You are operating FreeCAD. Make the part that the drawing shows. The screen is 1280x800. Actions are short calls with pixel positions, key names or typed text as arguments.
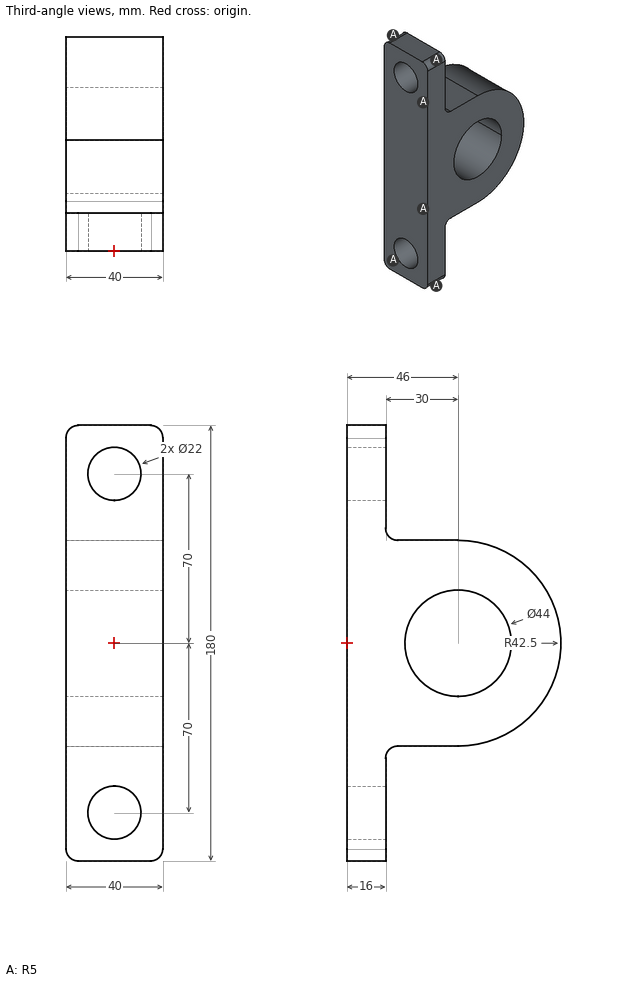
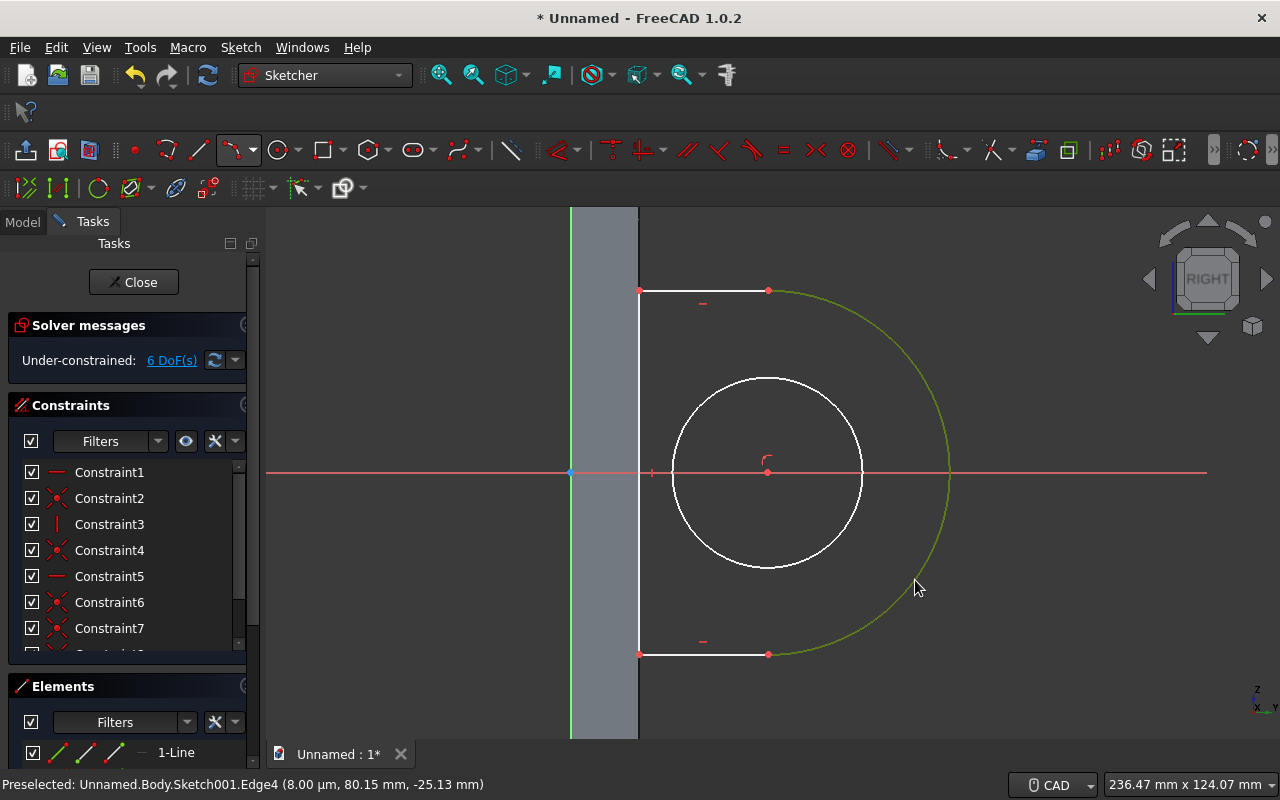
key(k)
key(r)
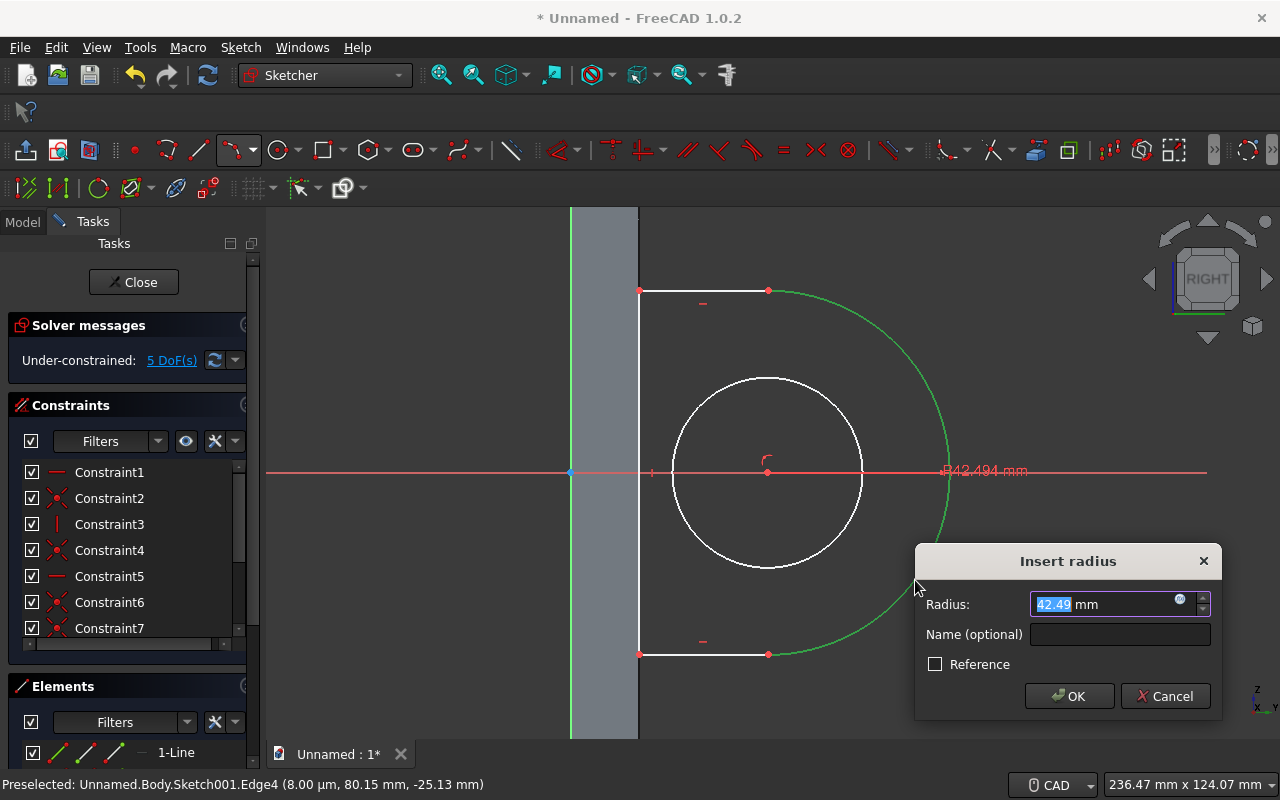
text(42.5)
key(Return)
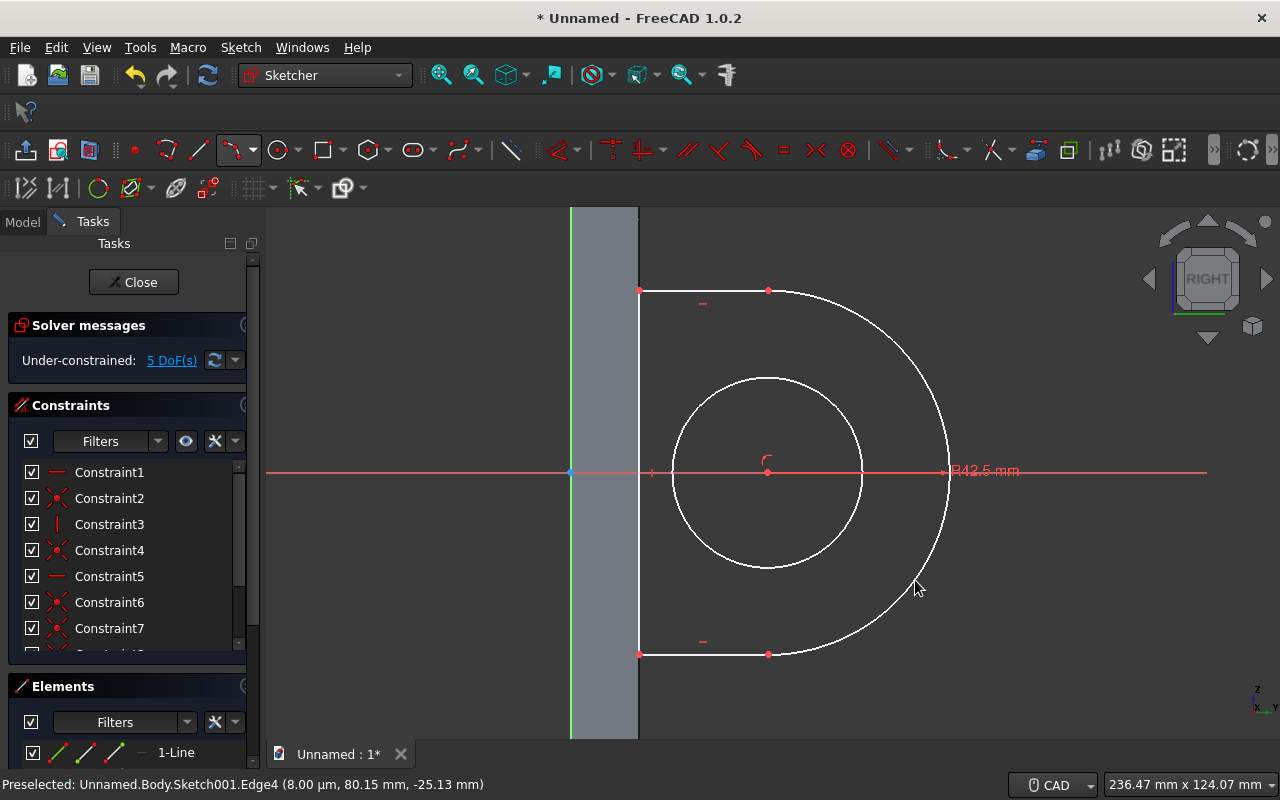
click(835, 405)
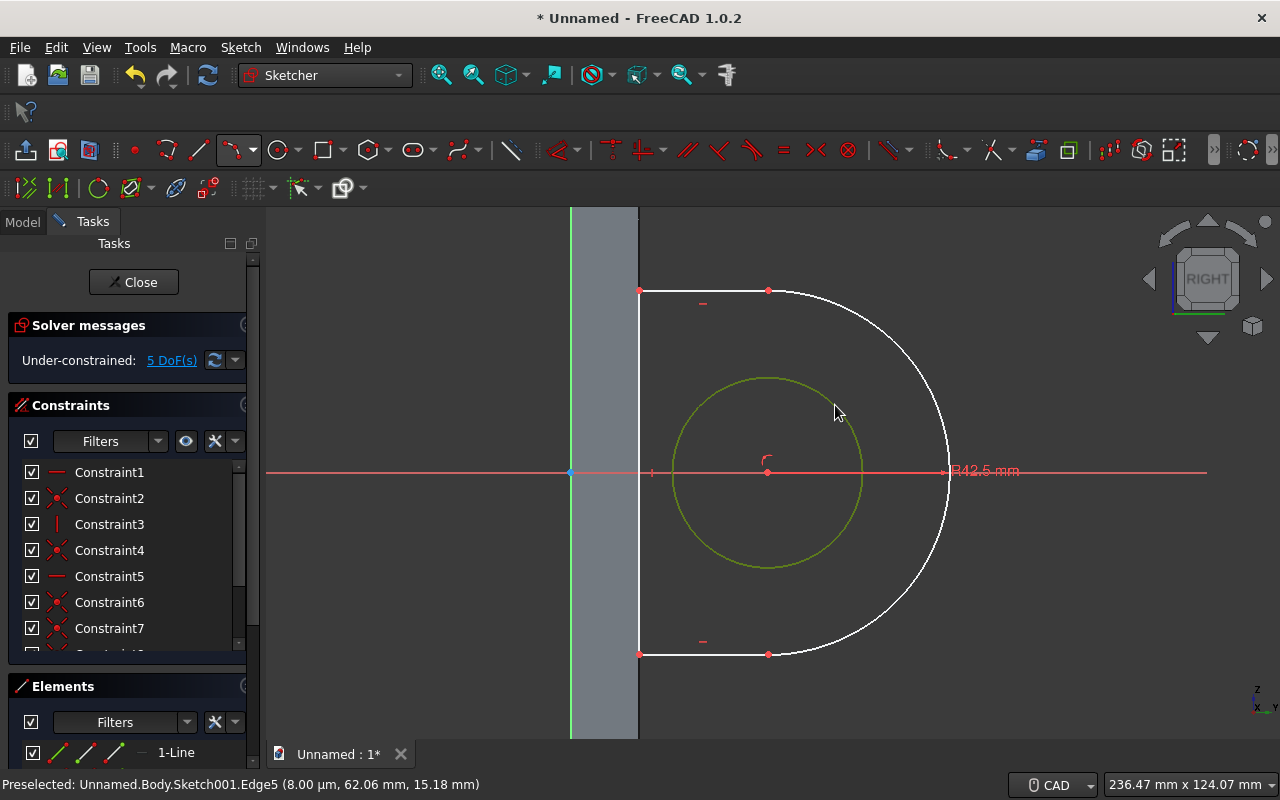
key(k)
key(o)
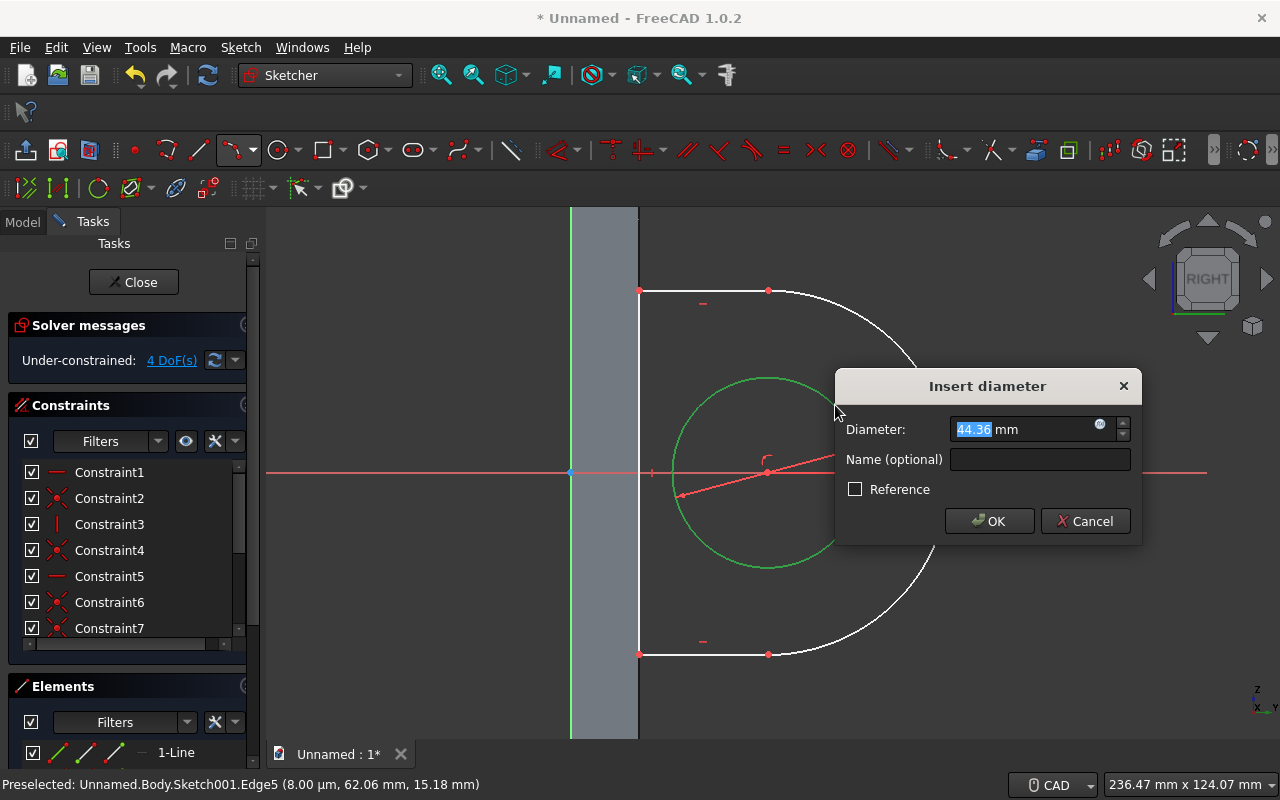
text(44)
key(Return)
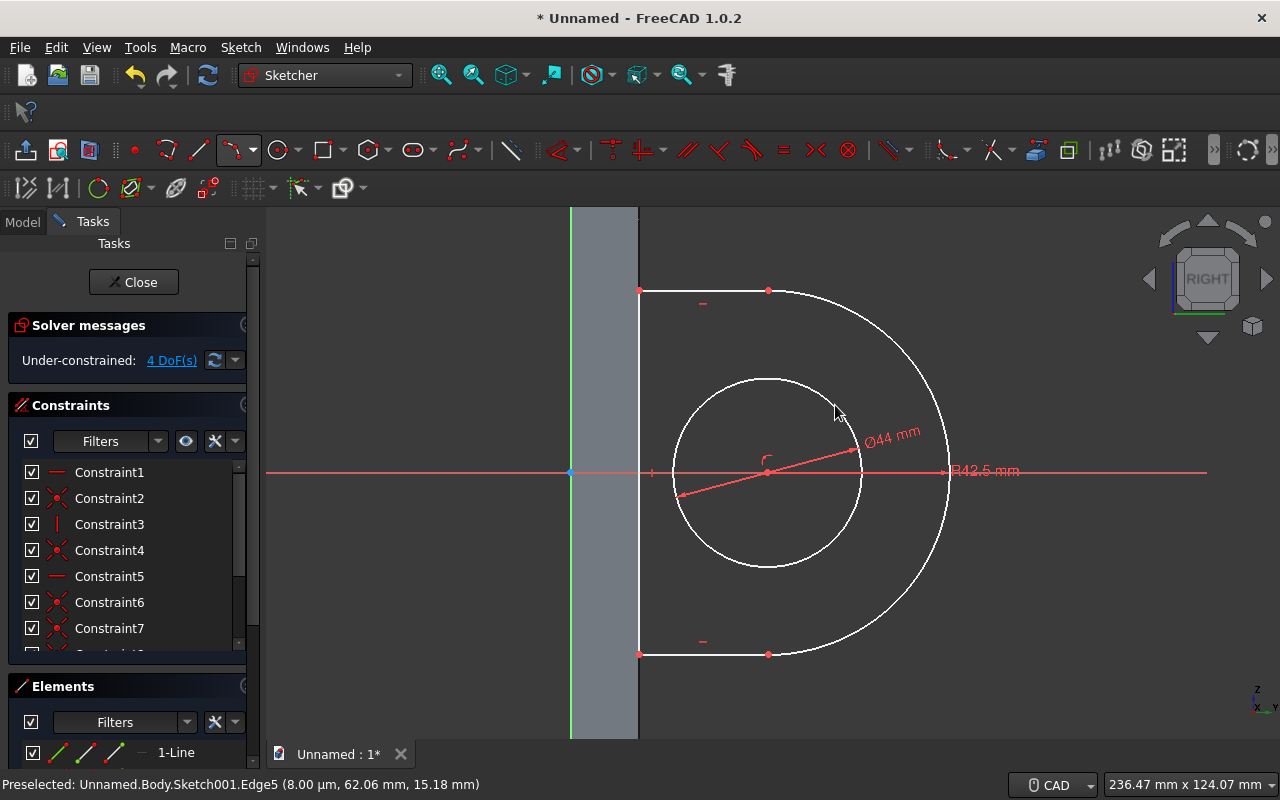
click(729, 291)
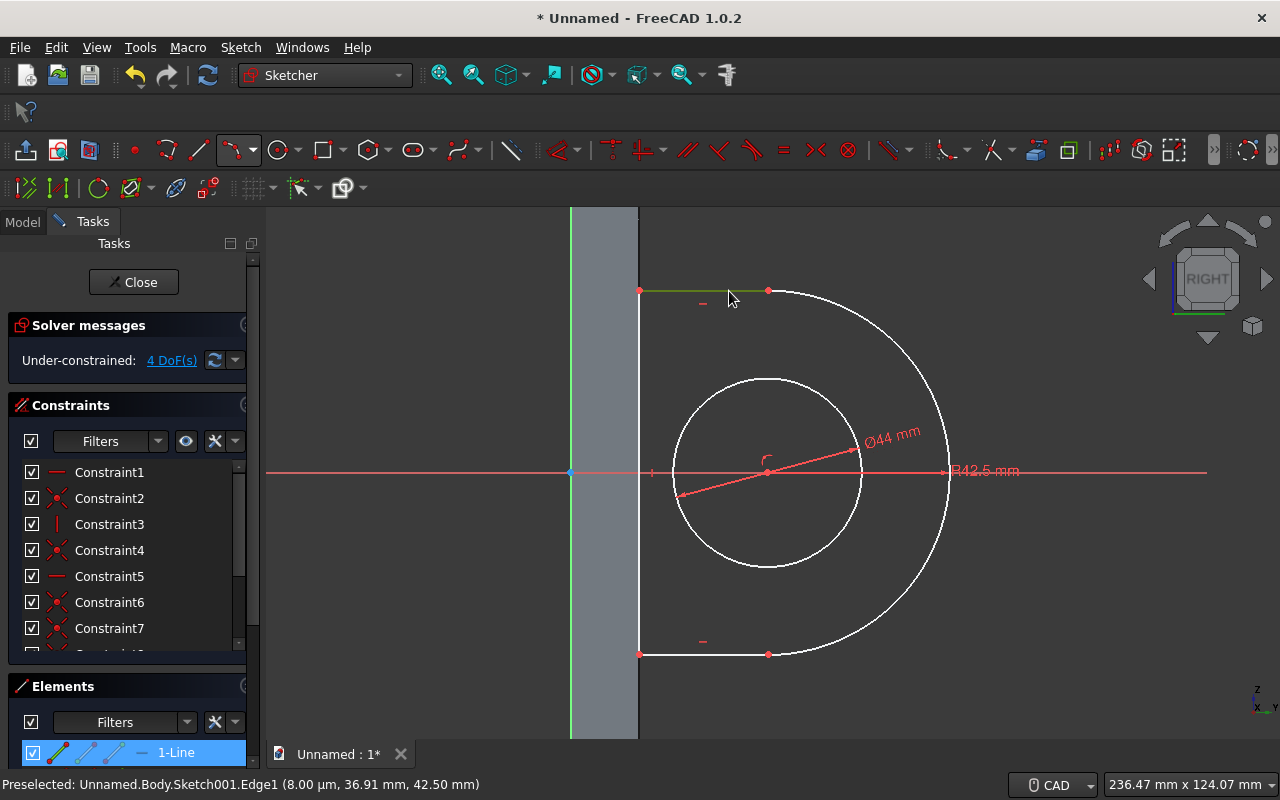
key(l)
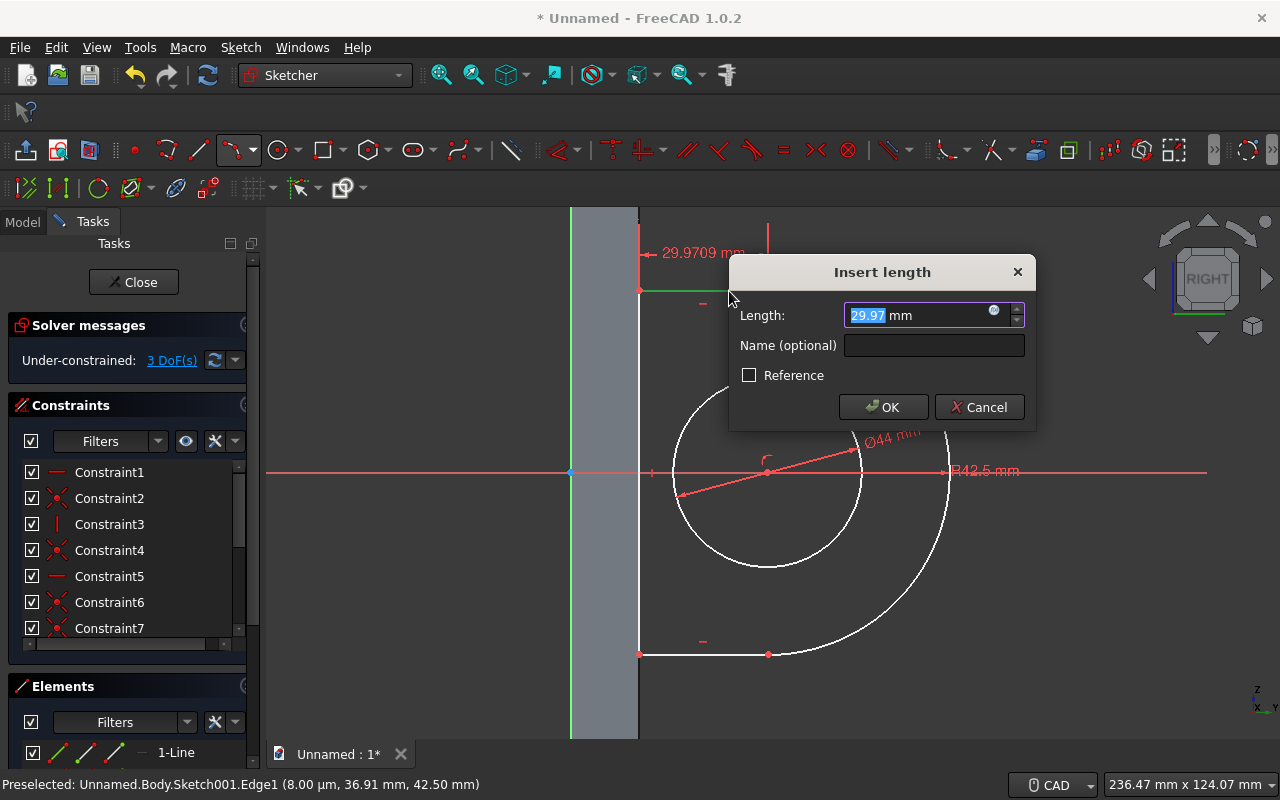
text(30)
key(Return)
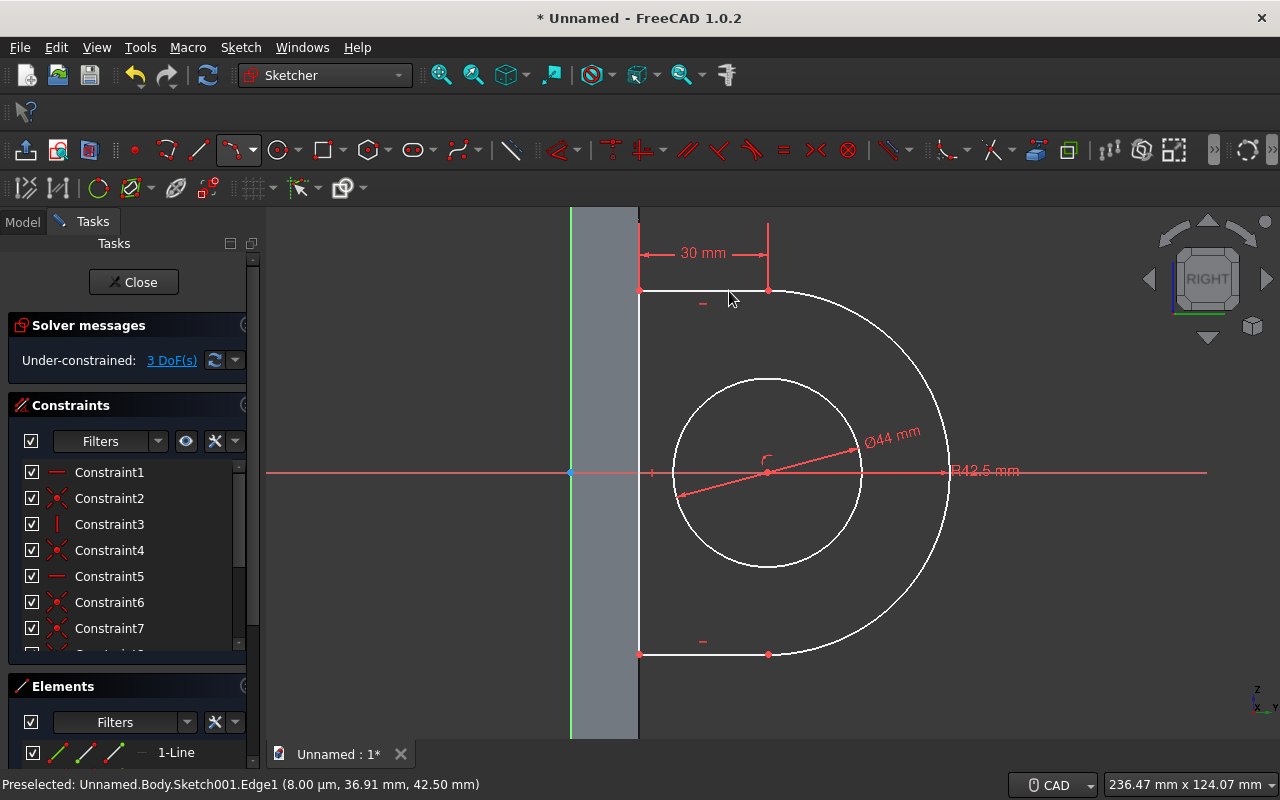
click(678, 655)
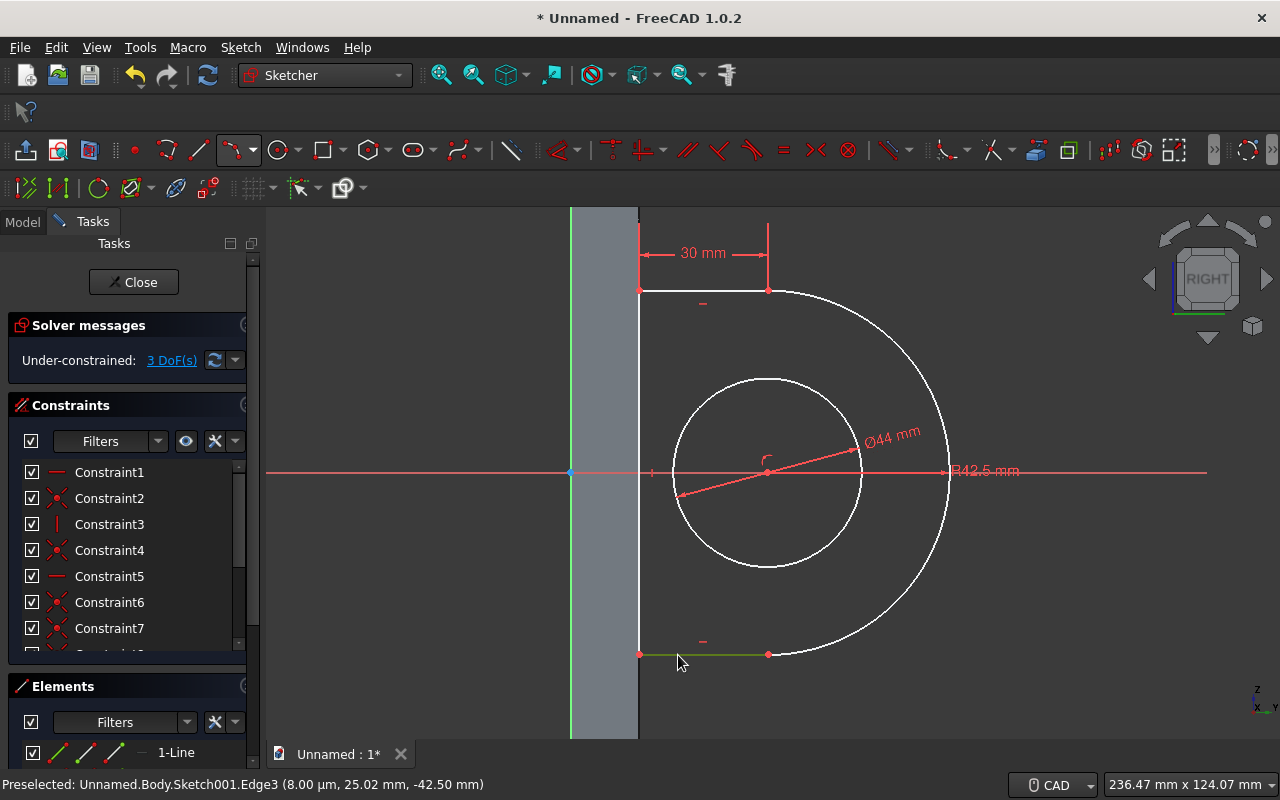
key(l)